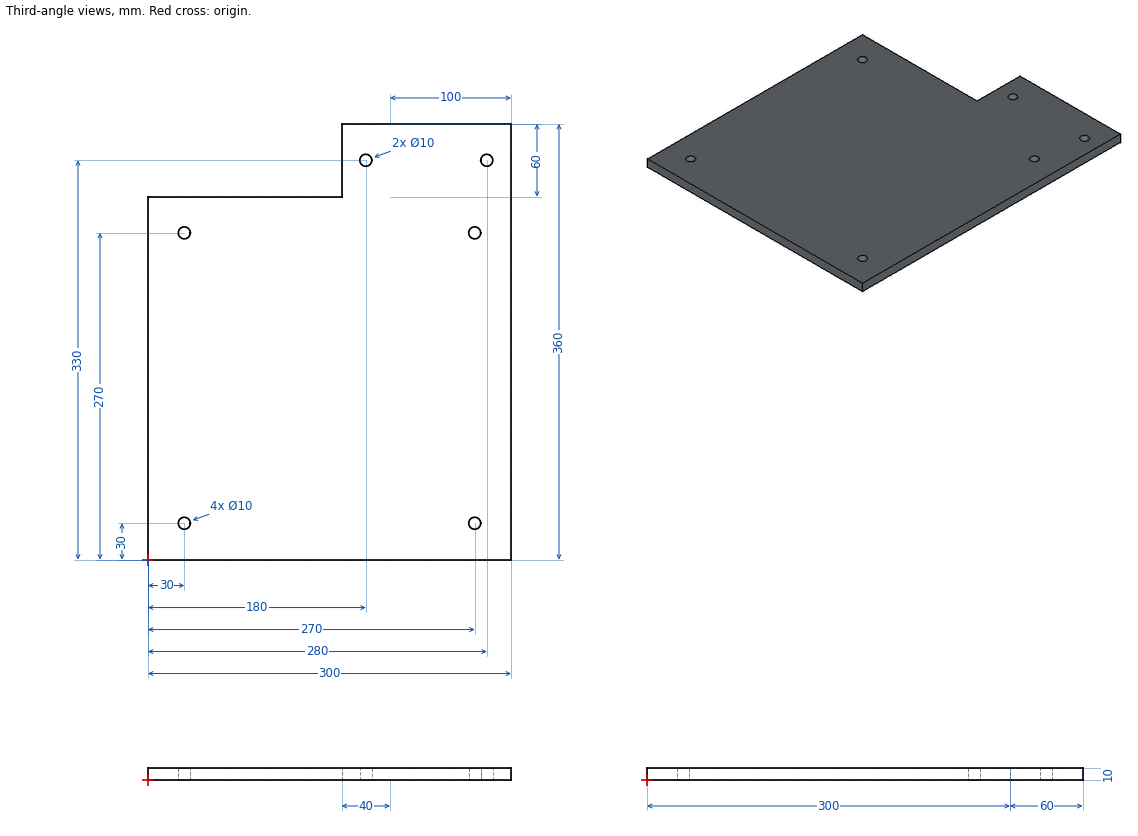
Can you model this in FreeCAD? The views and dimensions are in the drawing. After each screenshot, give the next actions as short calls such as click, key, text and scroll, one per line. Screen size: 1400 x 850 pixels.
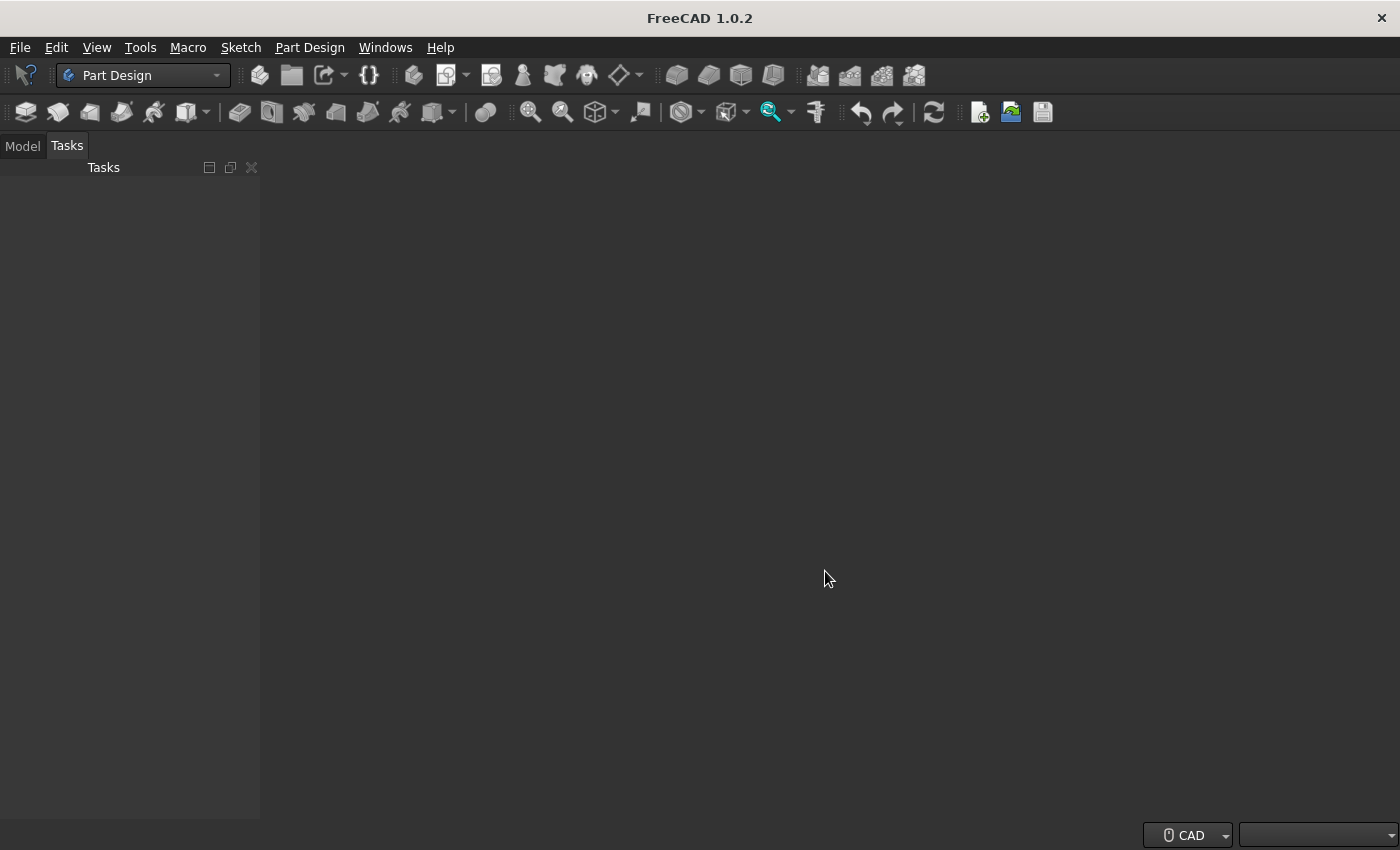
click(980, 112)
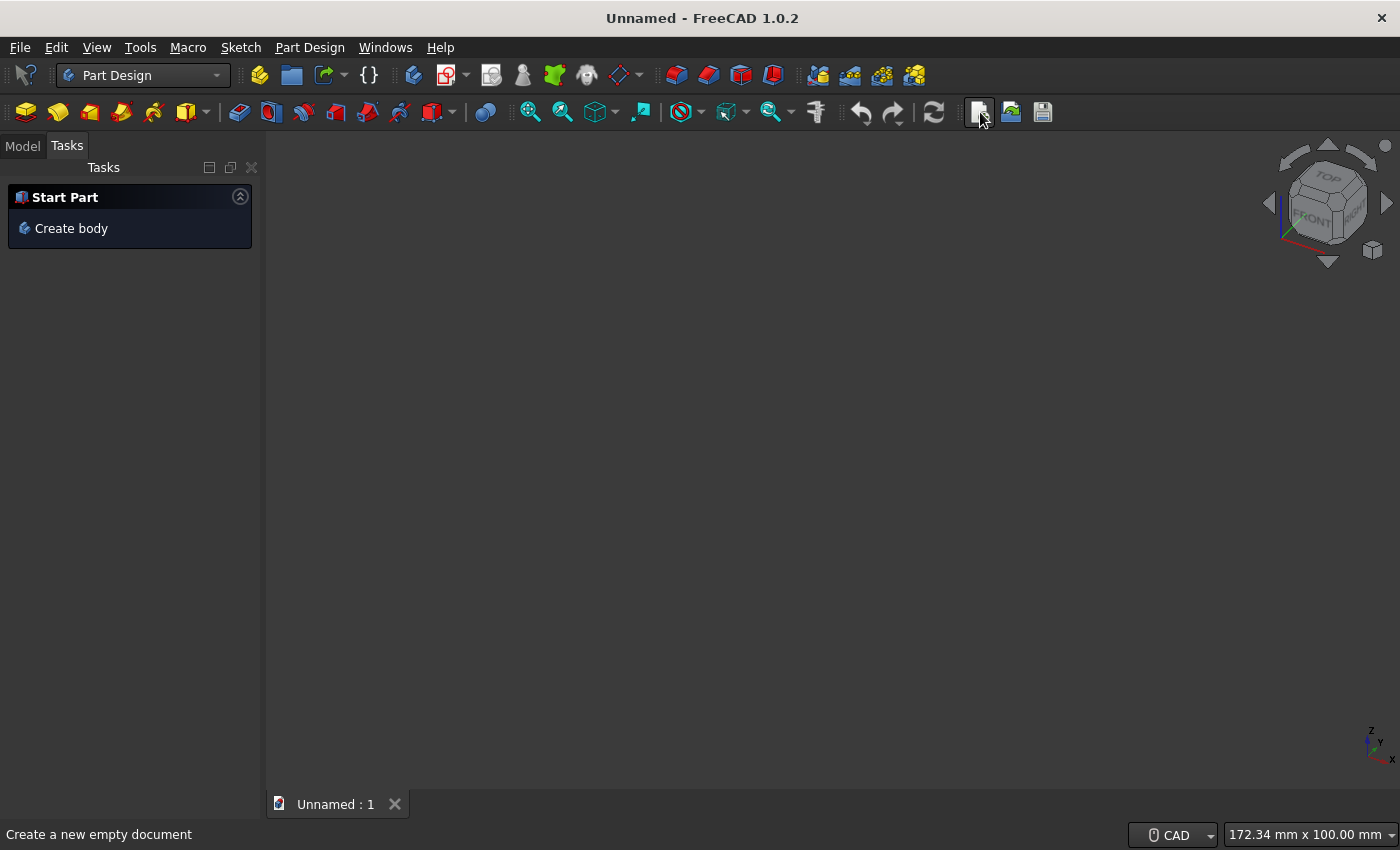
click(446, 76)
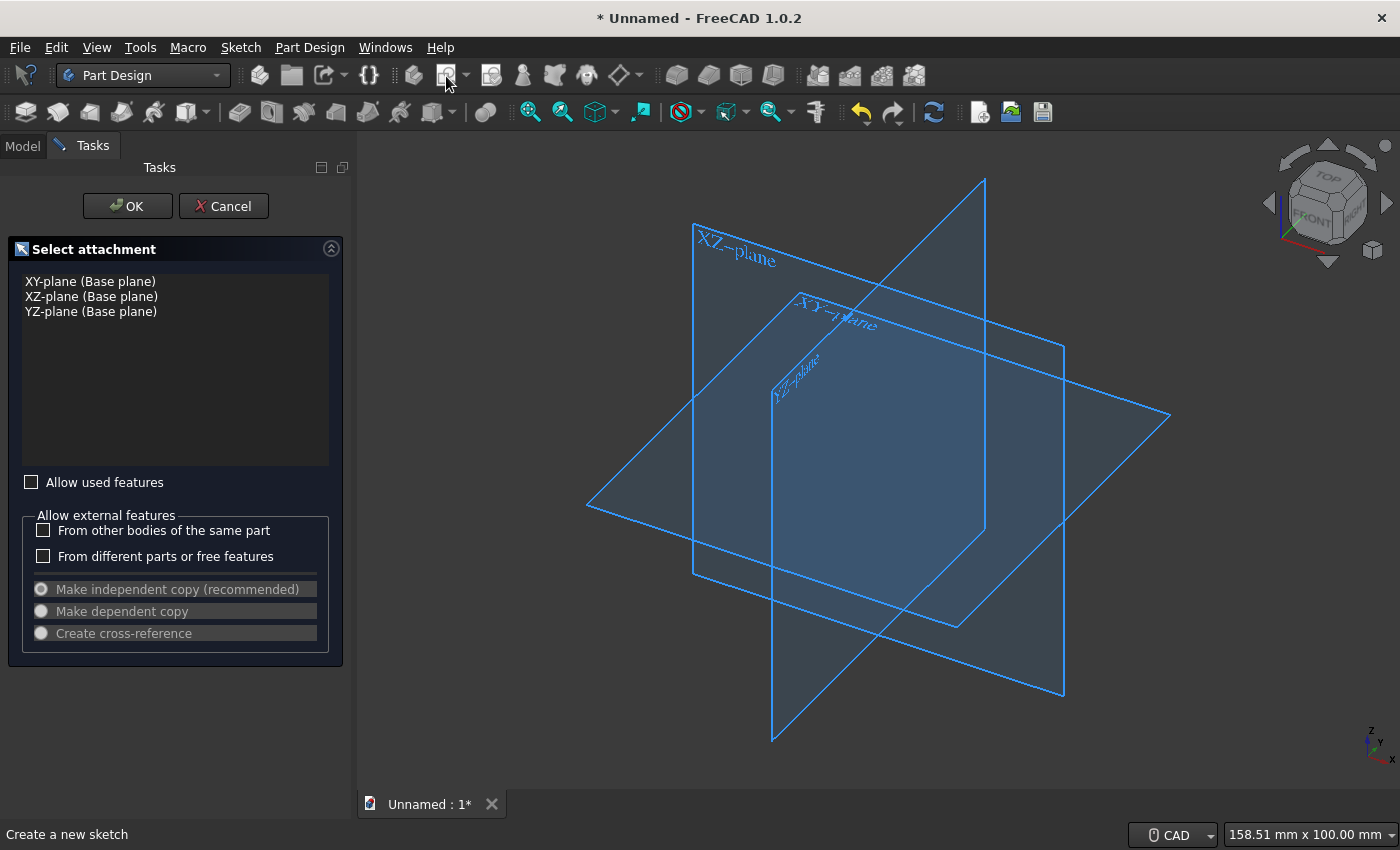
click(82, 282)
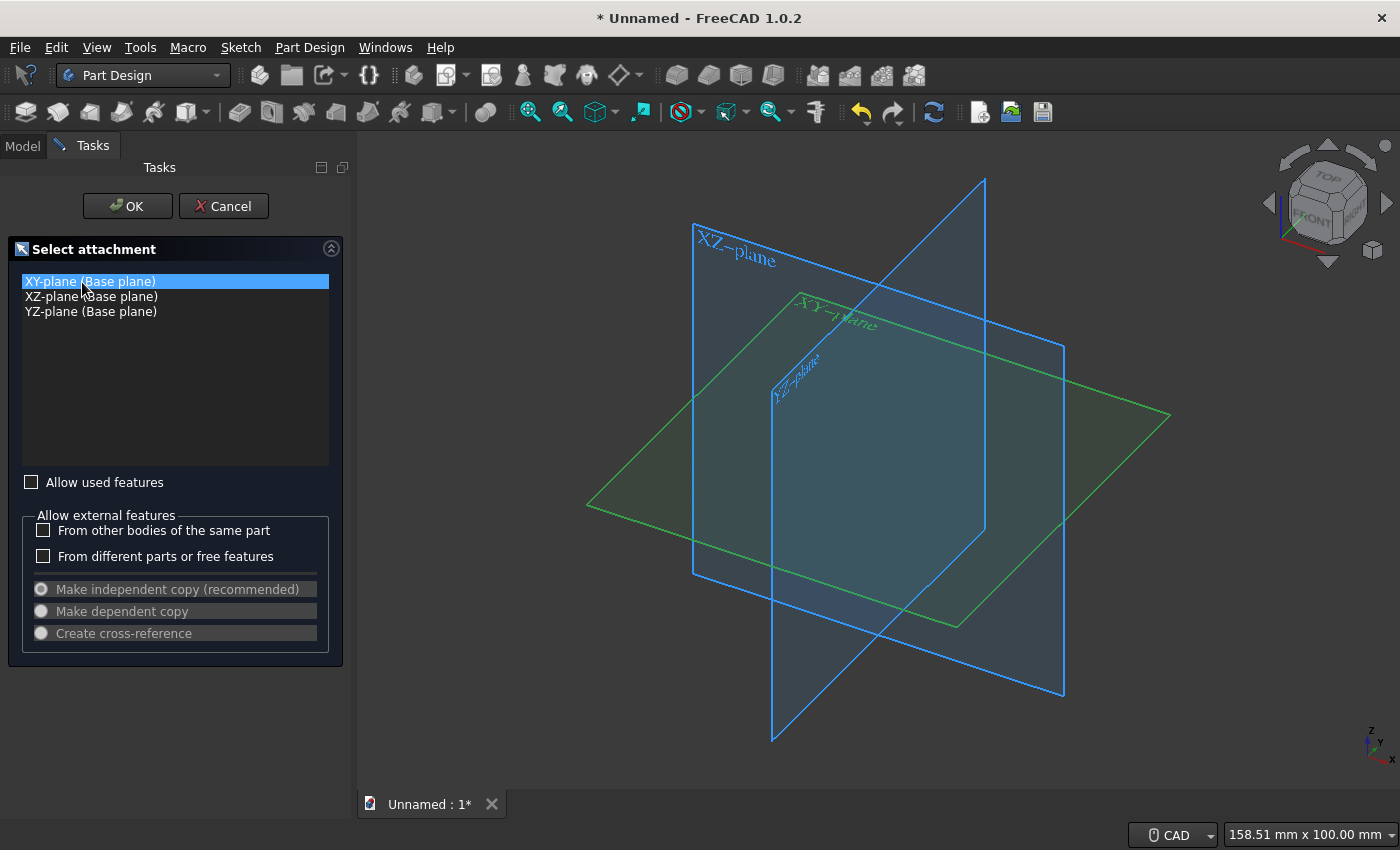
click(128, 206)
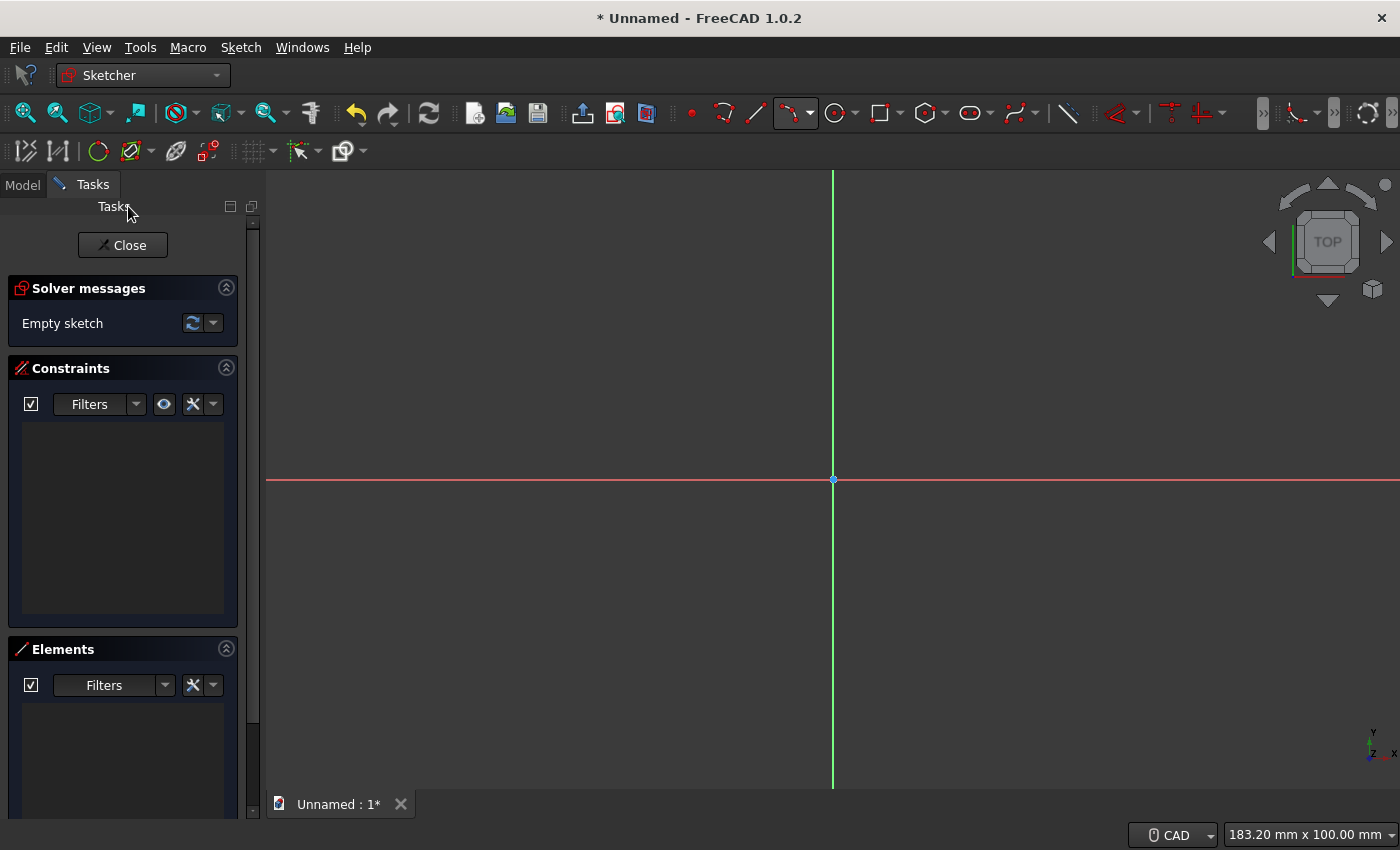
scroll(567, 700, down, 9)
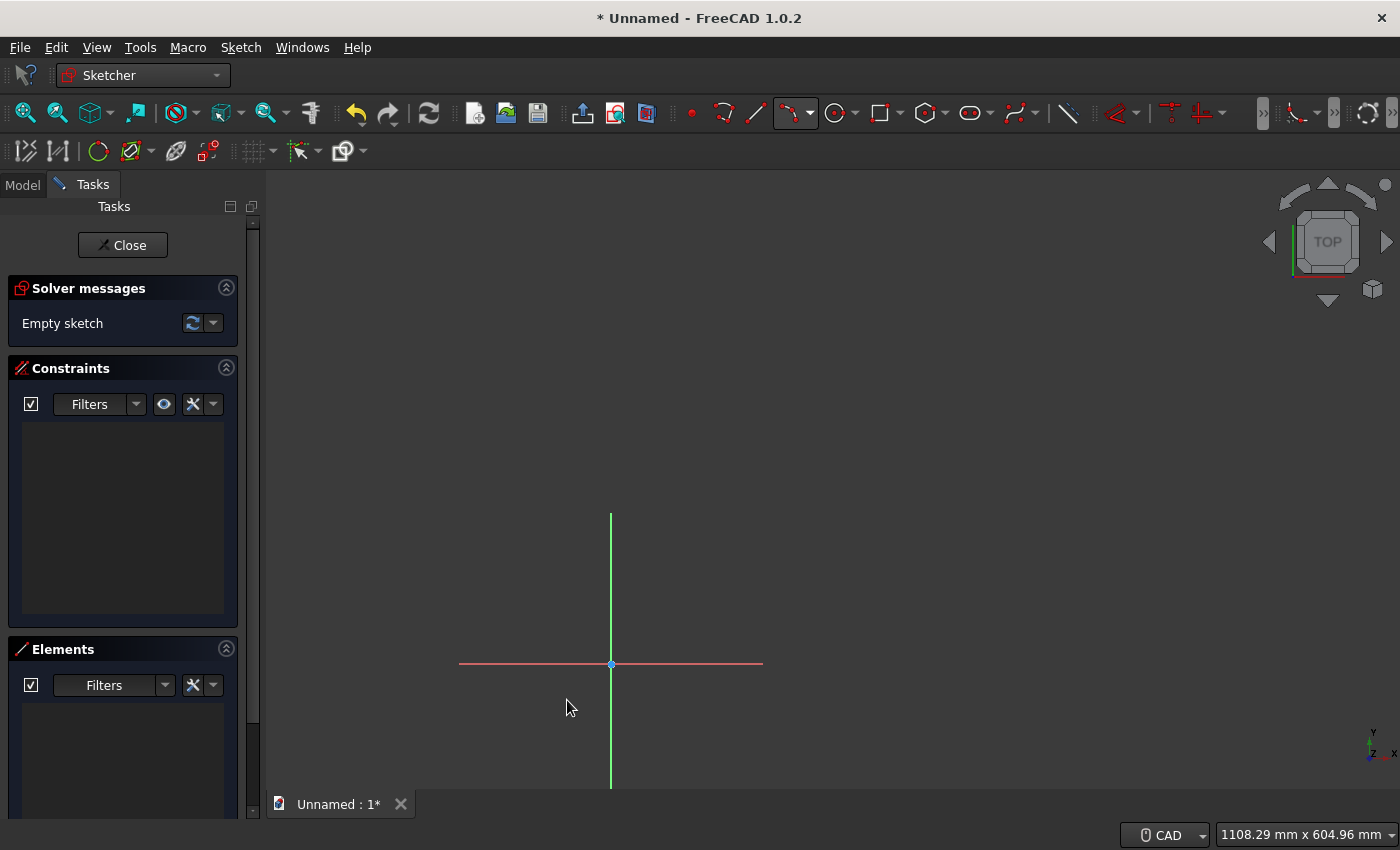
click(724, 114)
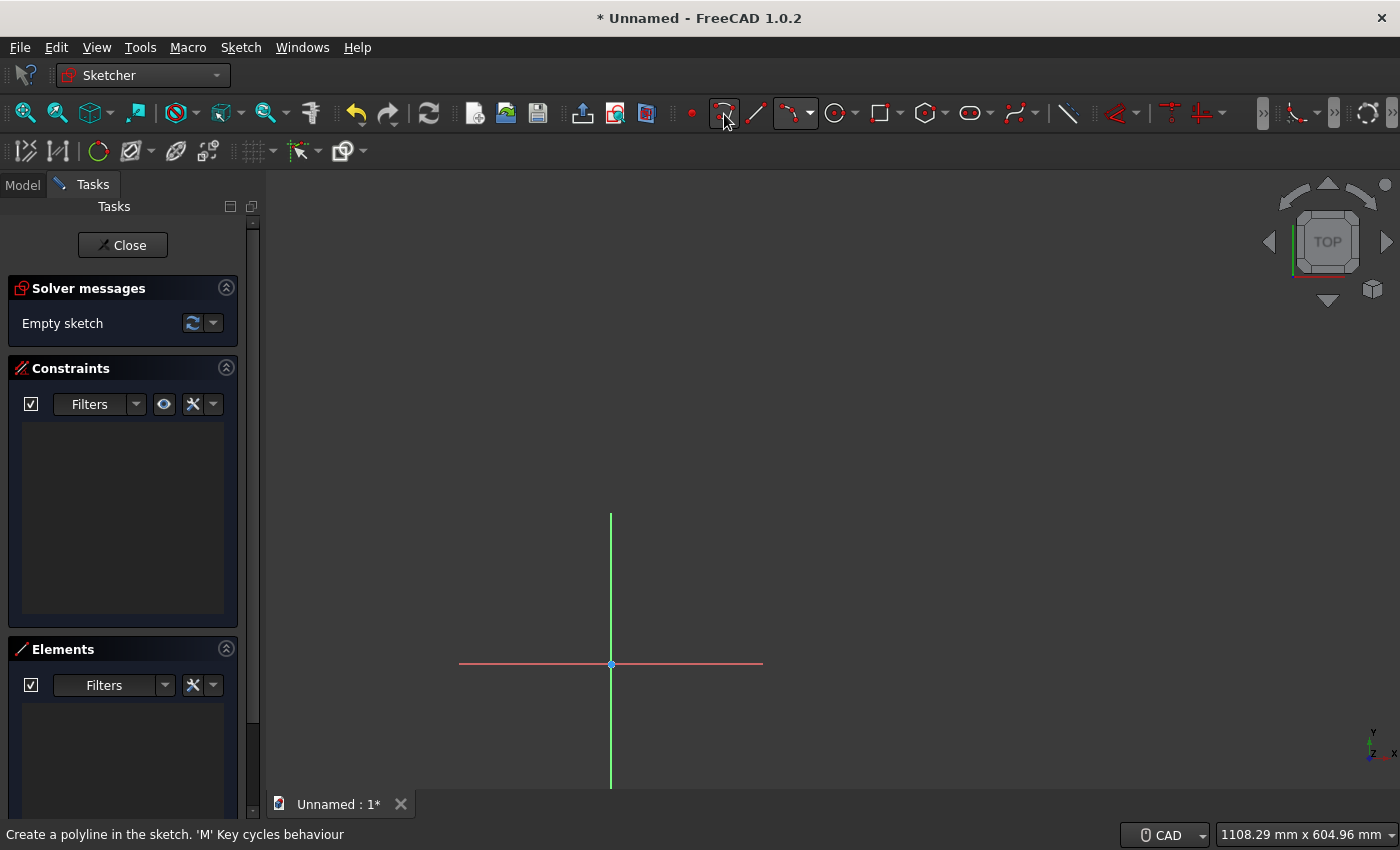
click(611, 664)
click(918, 655)
click(918, 296)
click(816, 296)
click(816, 357)
click(620, 357)
click(611, 664)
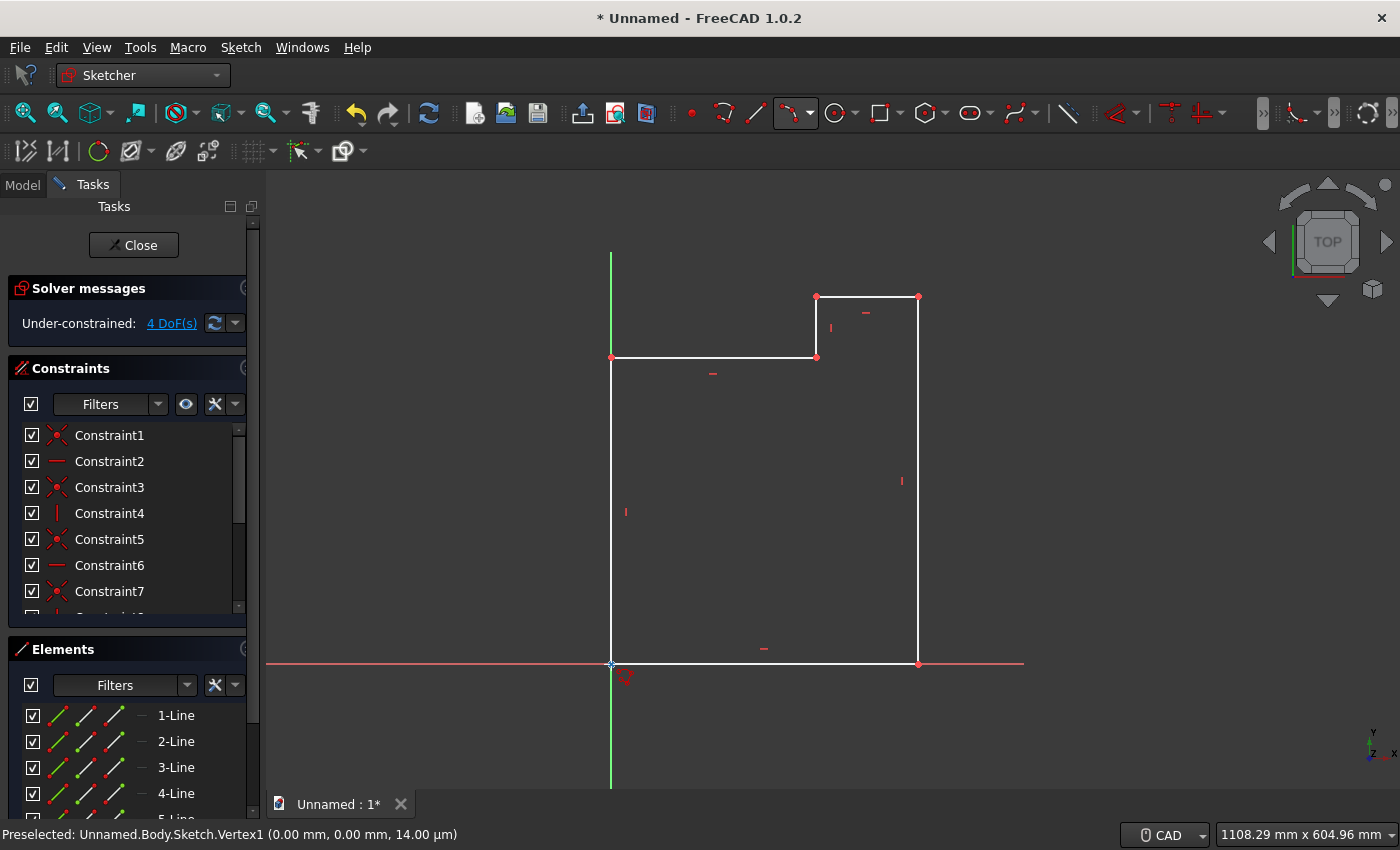
click(836, 114)